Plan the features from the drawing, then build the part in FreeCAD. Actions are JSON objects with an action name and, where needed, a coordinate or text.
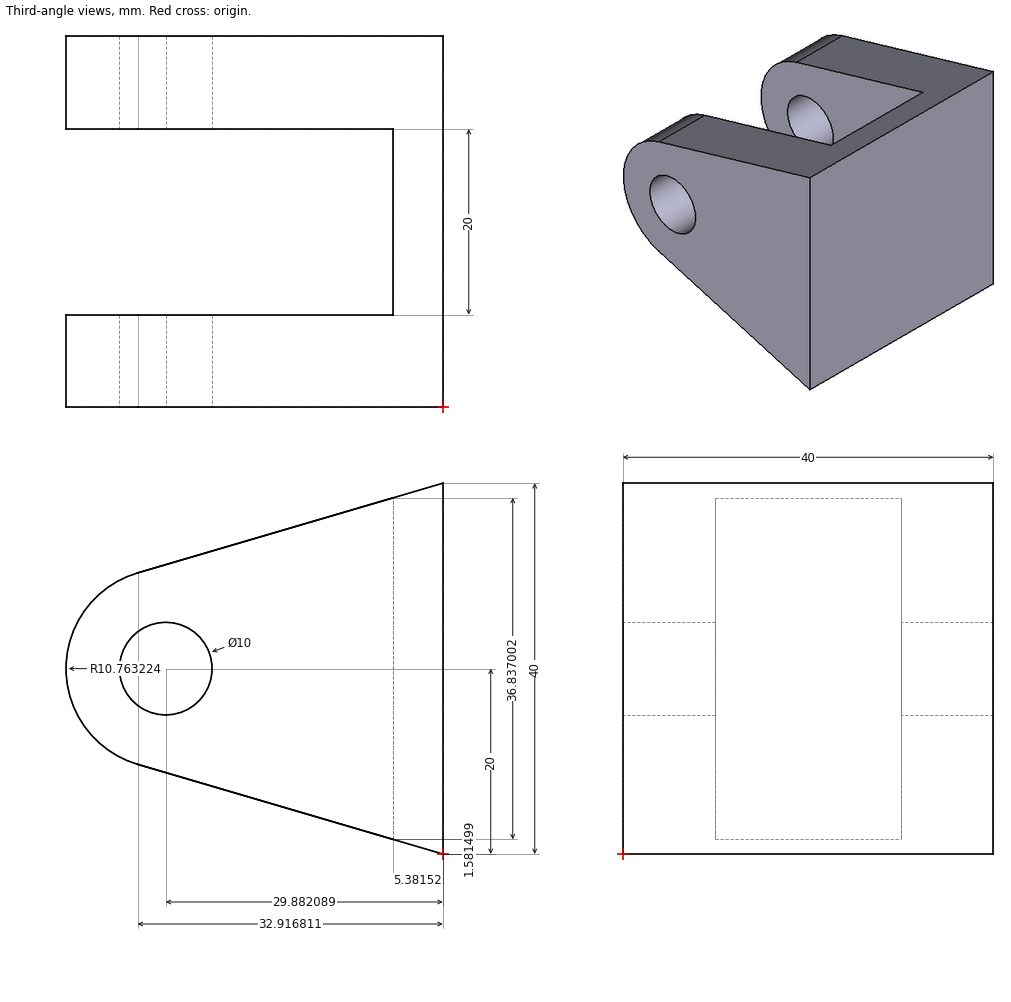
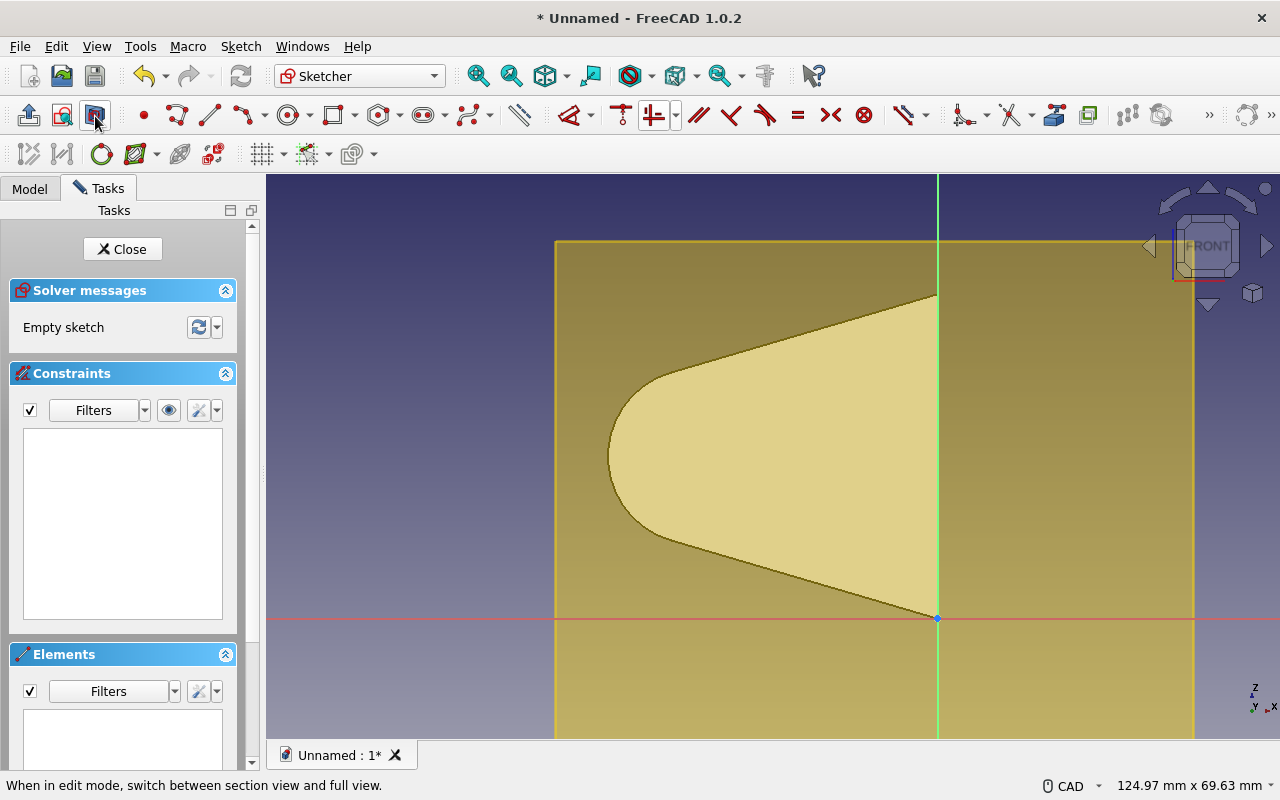
{"action": "left_click", "coordinate": [177, 116]}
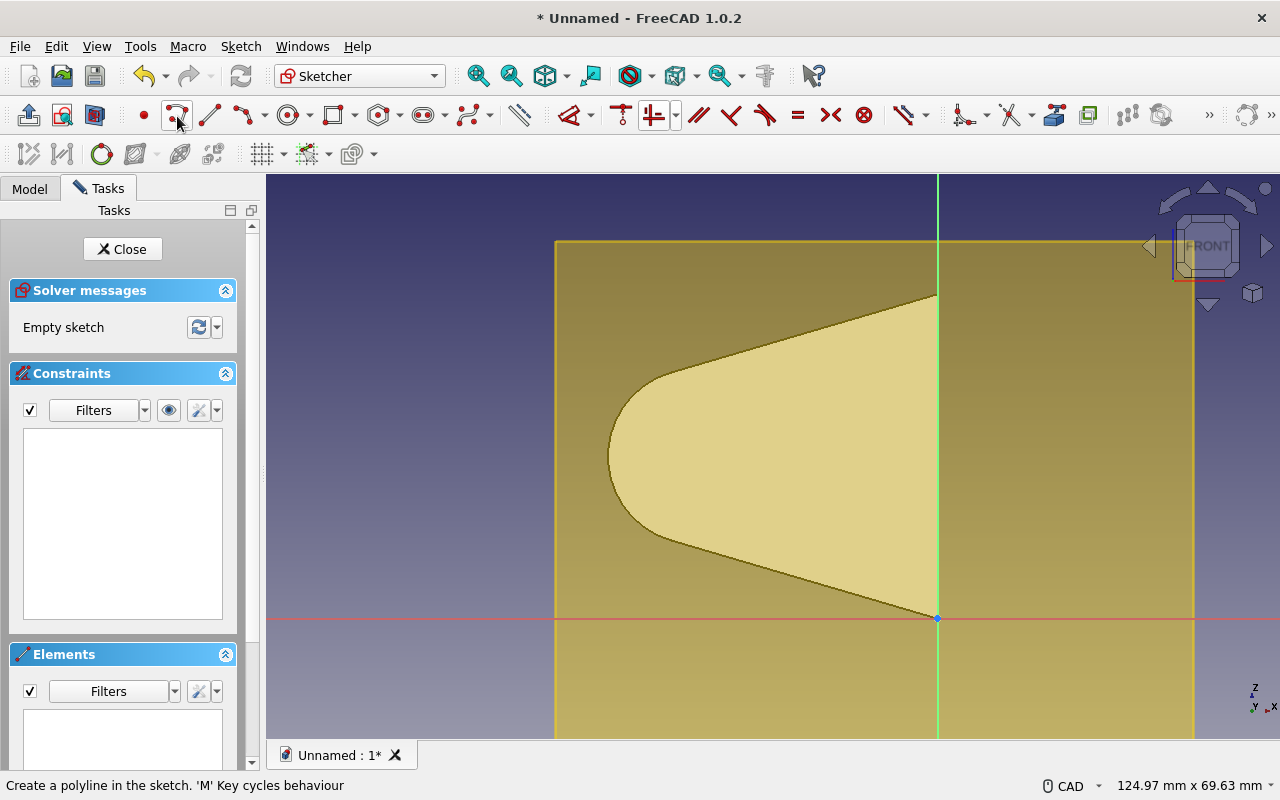
{"action": "left_click", "coordinate": [671, 540]}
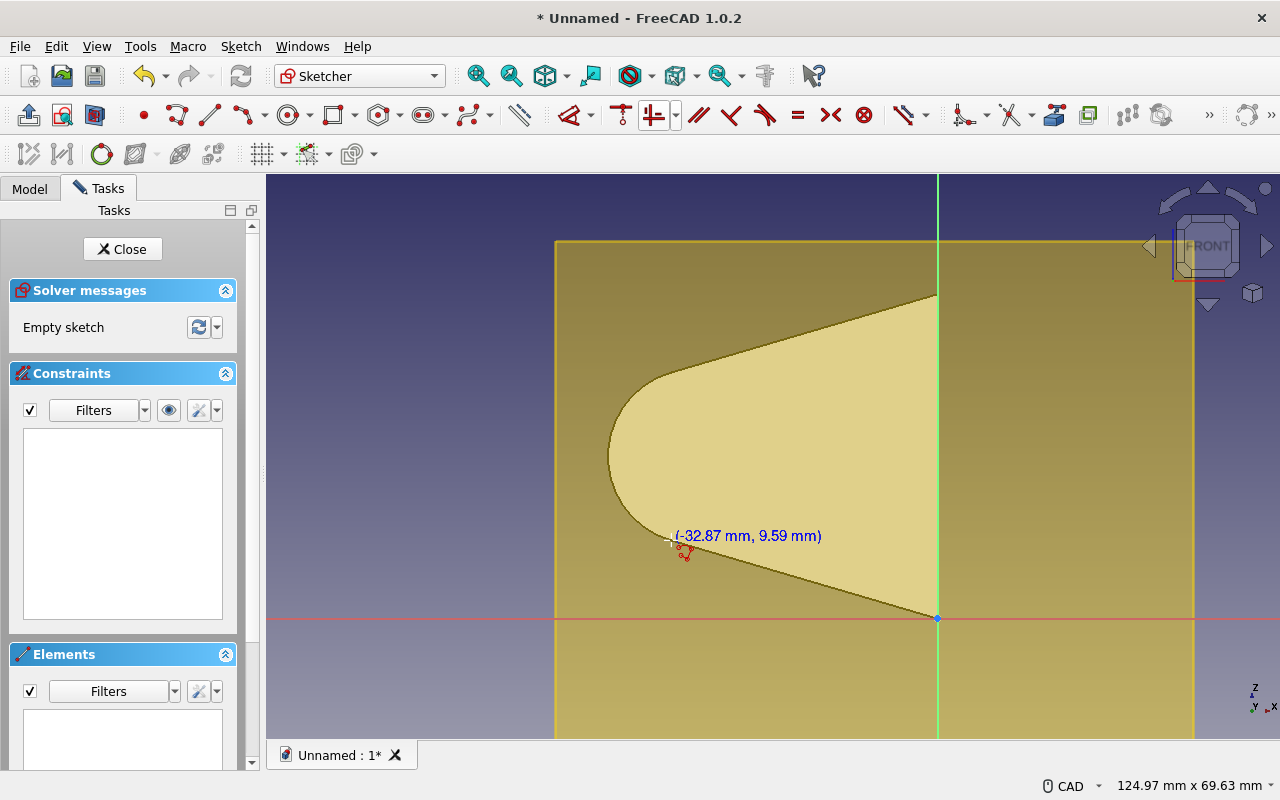
{"action": "scroll", "coordinate": [894, 606], "scroll_direction": "up", "scroll_amount": 2}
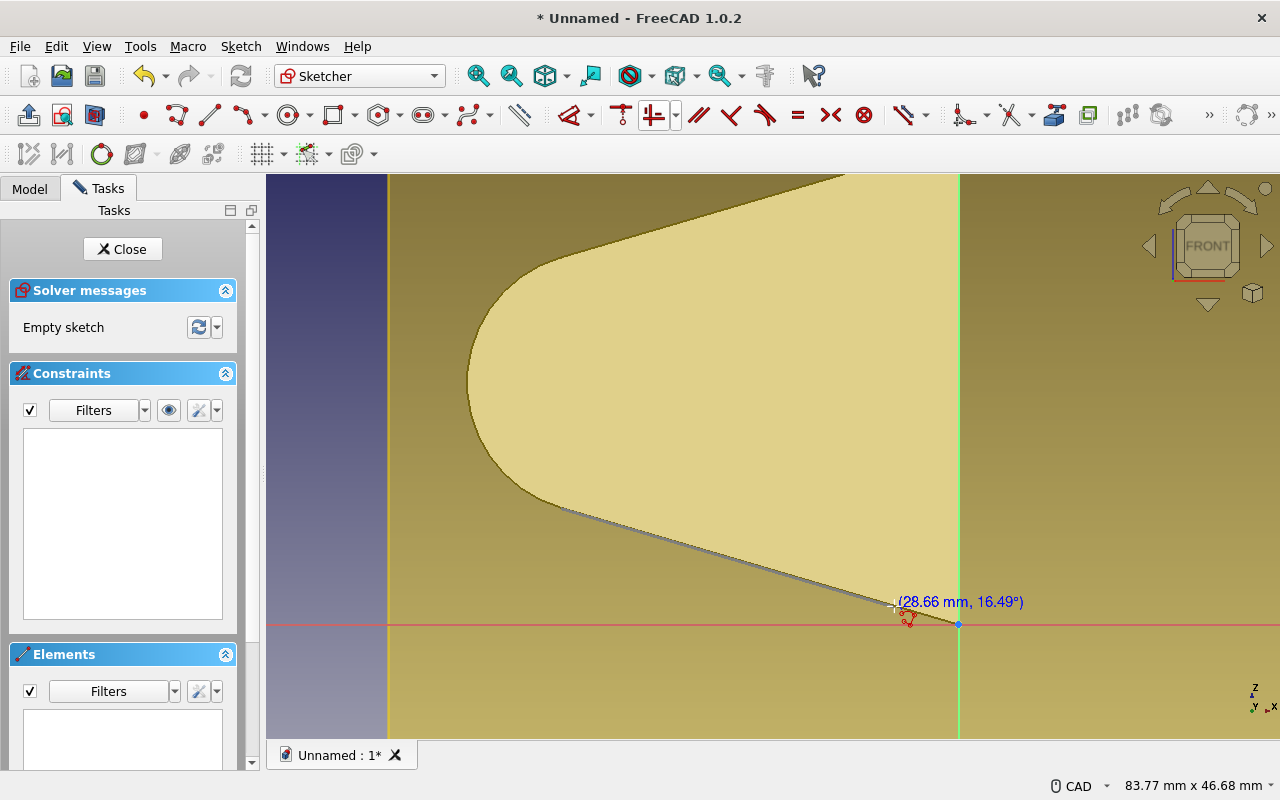
{"action": "left_click", "coordinate": [894, 606]}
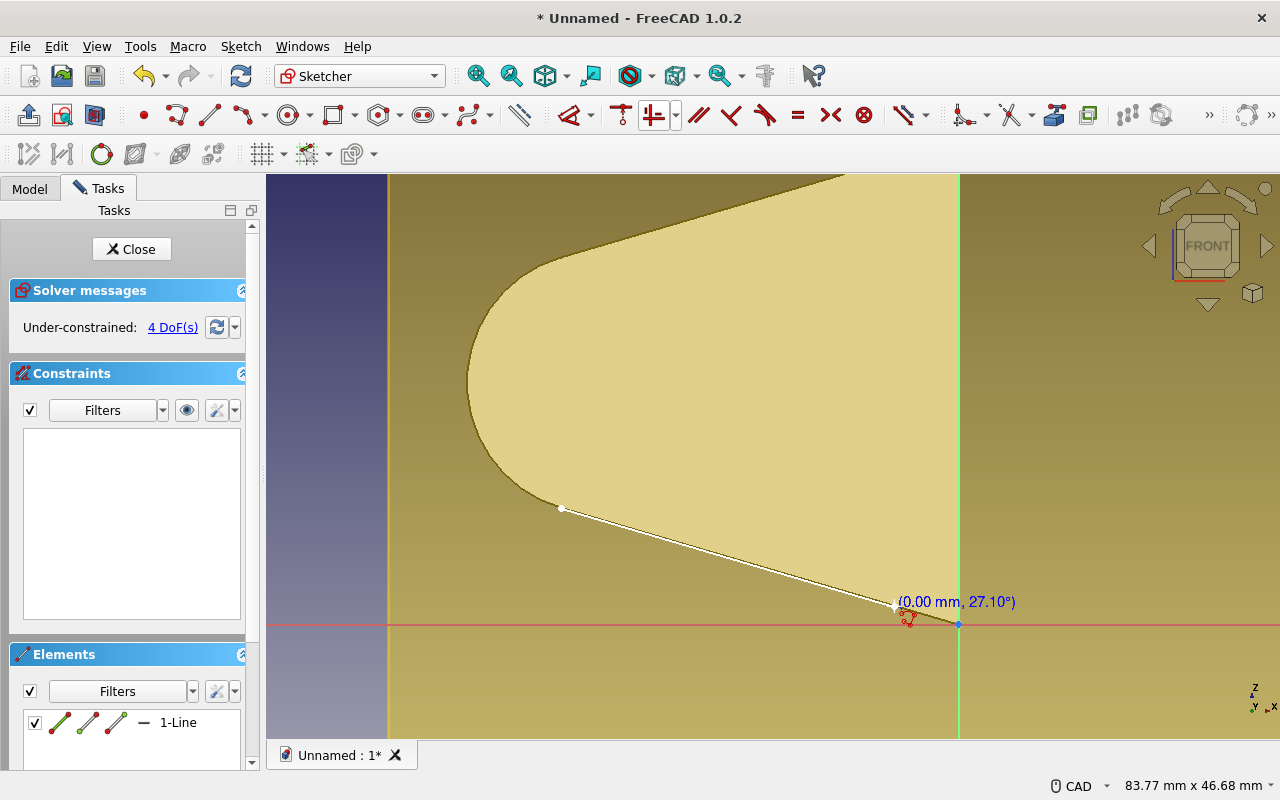
{"action": "scroll", "coordinate": [666, 711], "scroll_direction": "down", "scroll_amount": 1}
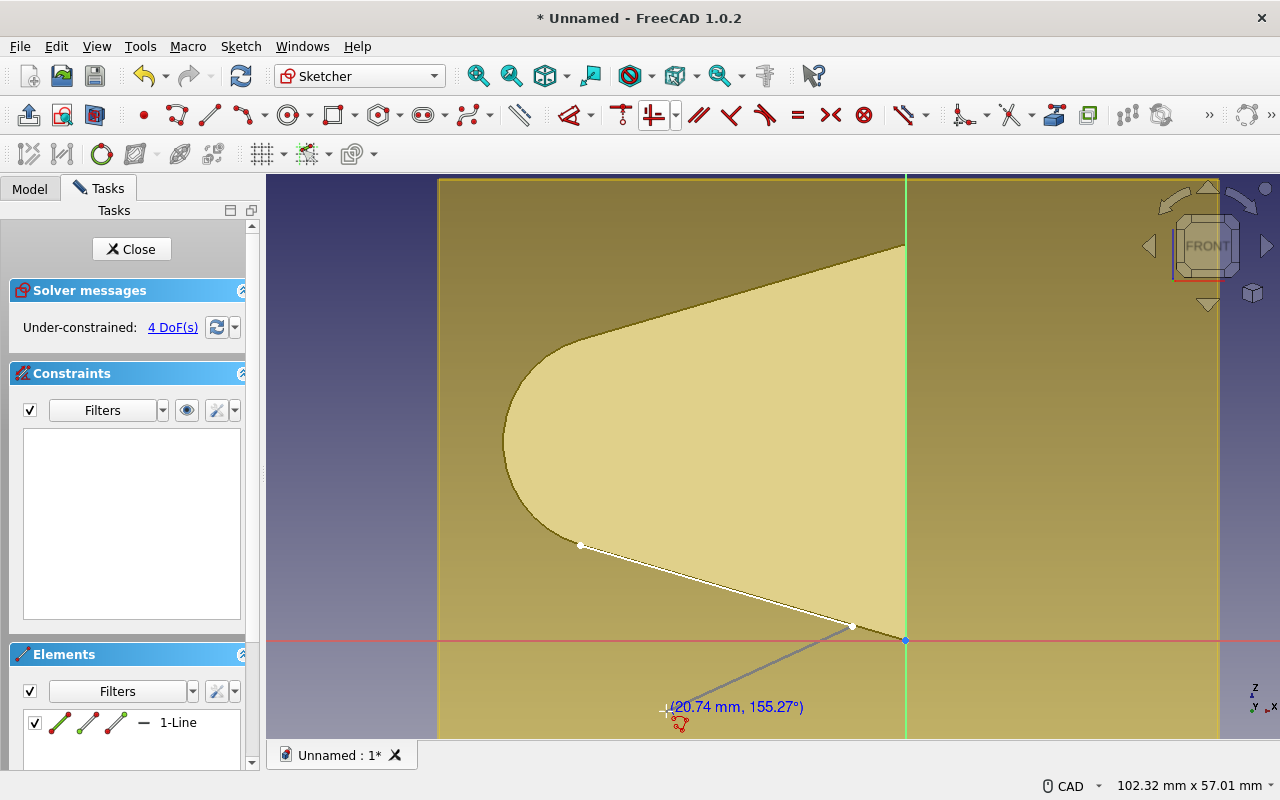
{"action": "left_click", "coordinate": [853, 260]}
{"action": "left_click", "coordinate": [580, 340]}
{"action": "right_click", "coordinate": [580, 340]}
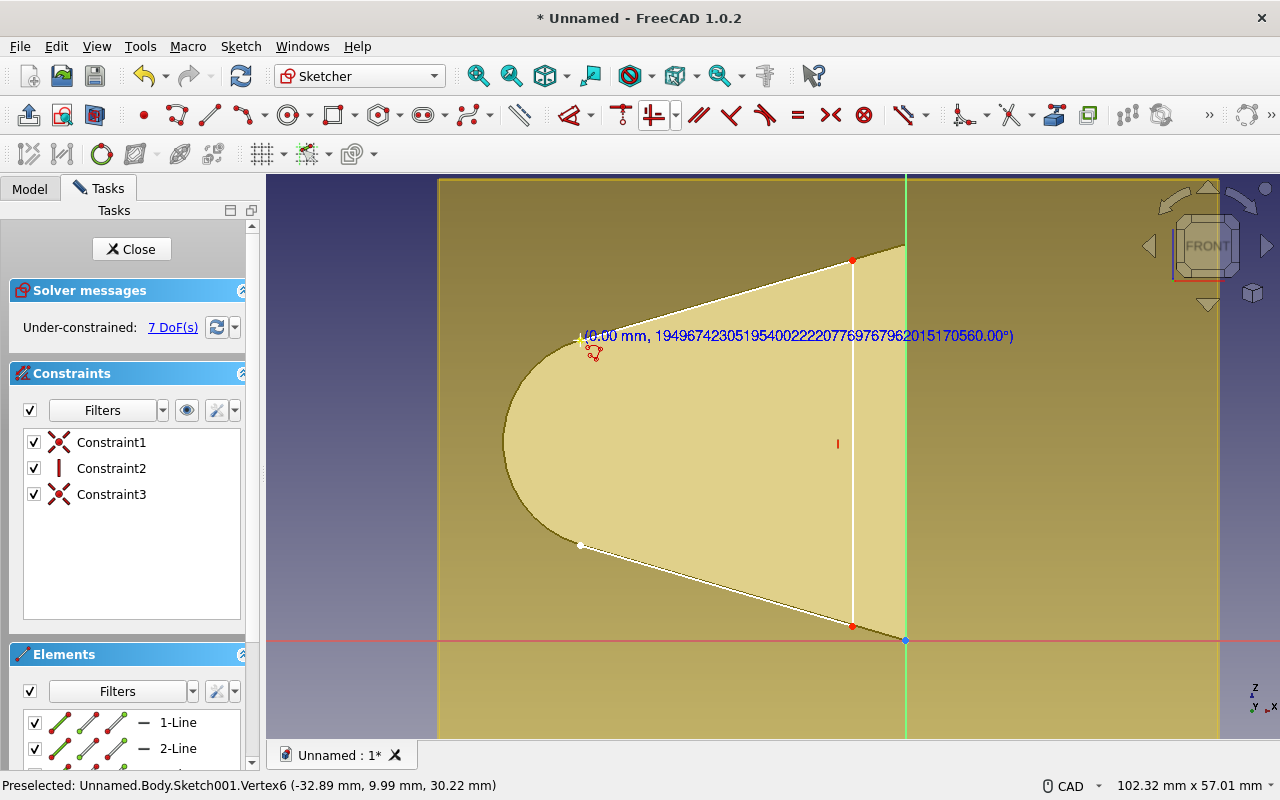
{"action": "left_click", "coordinate": [242, 116]}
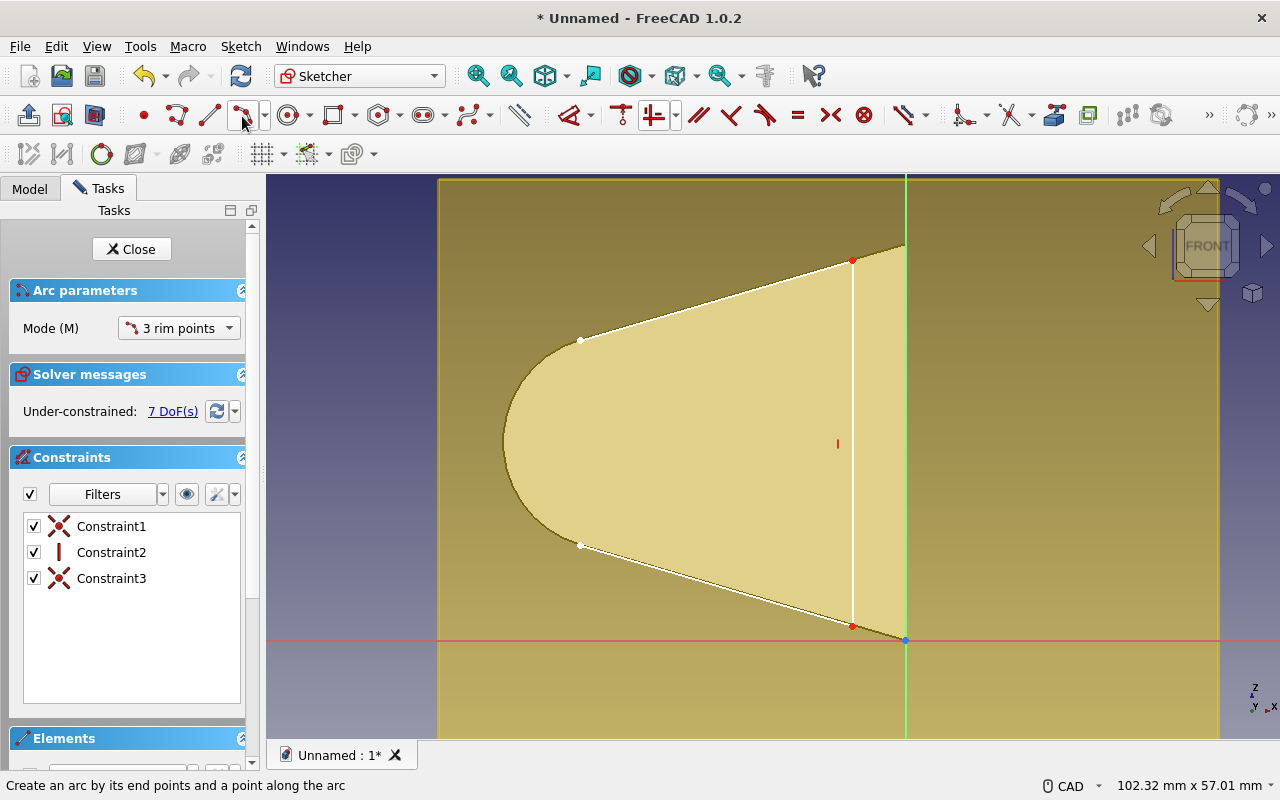
{"action": "left_click", "coordinate": [580, 341]}
{"action": "left_click", "coordinate": [580, 546]}
{"action": "left_click", "coordinate": [503, 442]}
{"action": "key", "text": "Escape"}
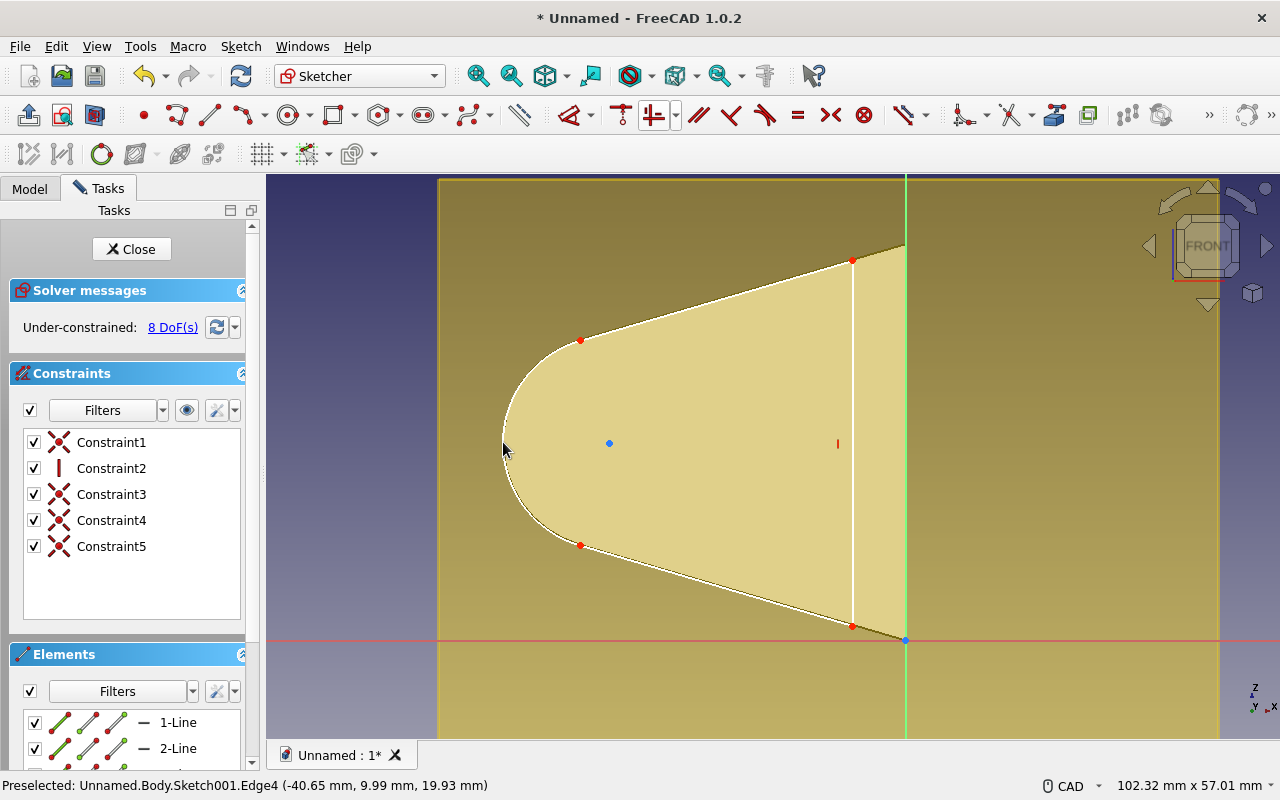
{"action": "left_click", "coordinate": [662, 570]}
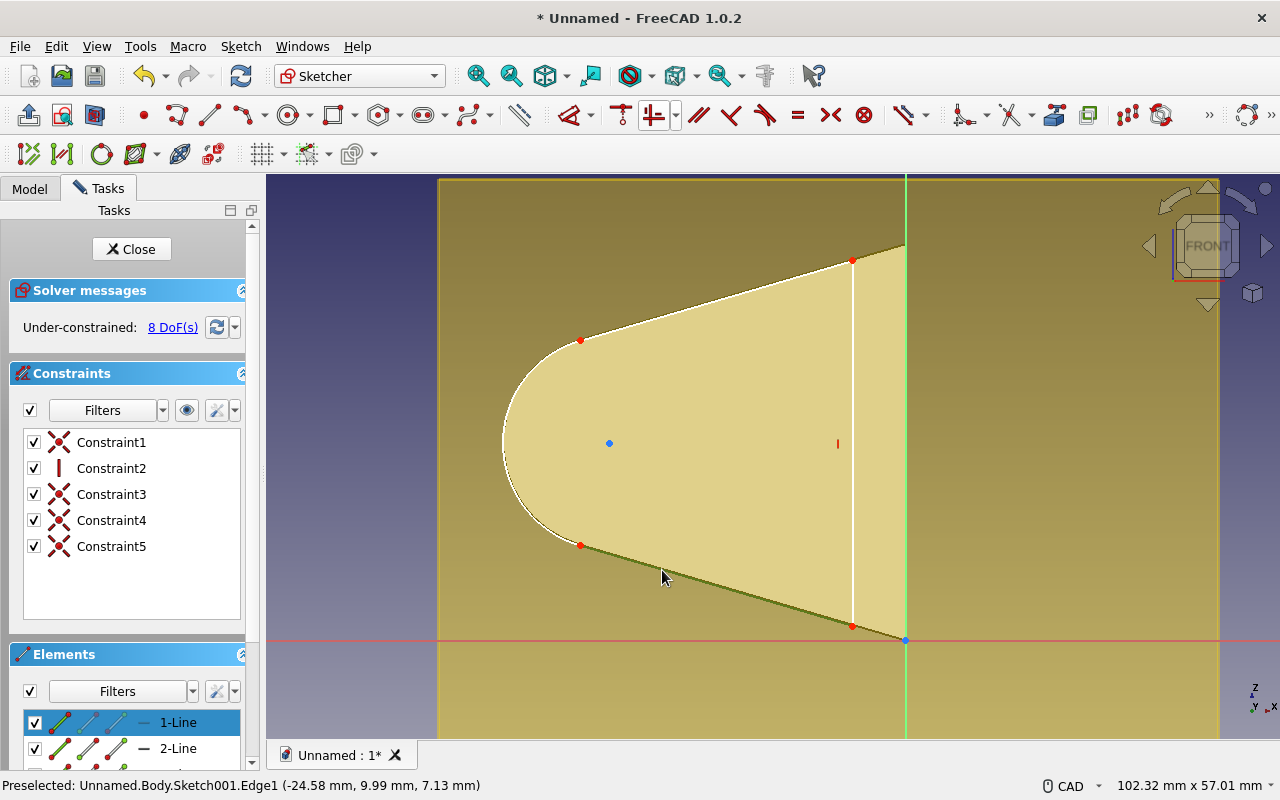
{"action": "left_click", "coordinate": [517, 391]}